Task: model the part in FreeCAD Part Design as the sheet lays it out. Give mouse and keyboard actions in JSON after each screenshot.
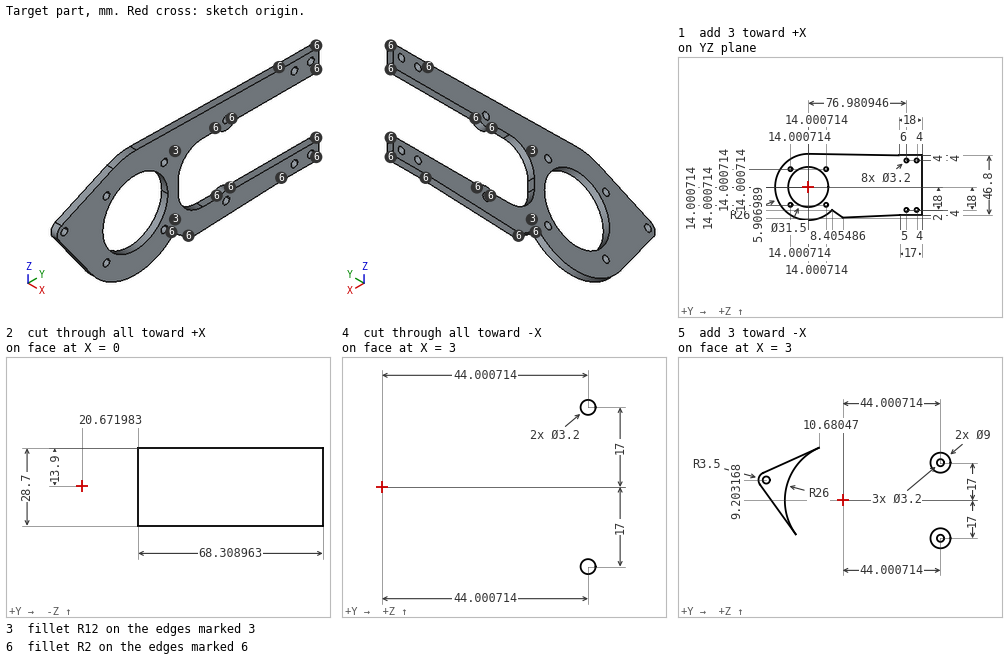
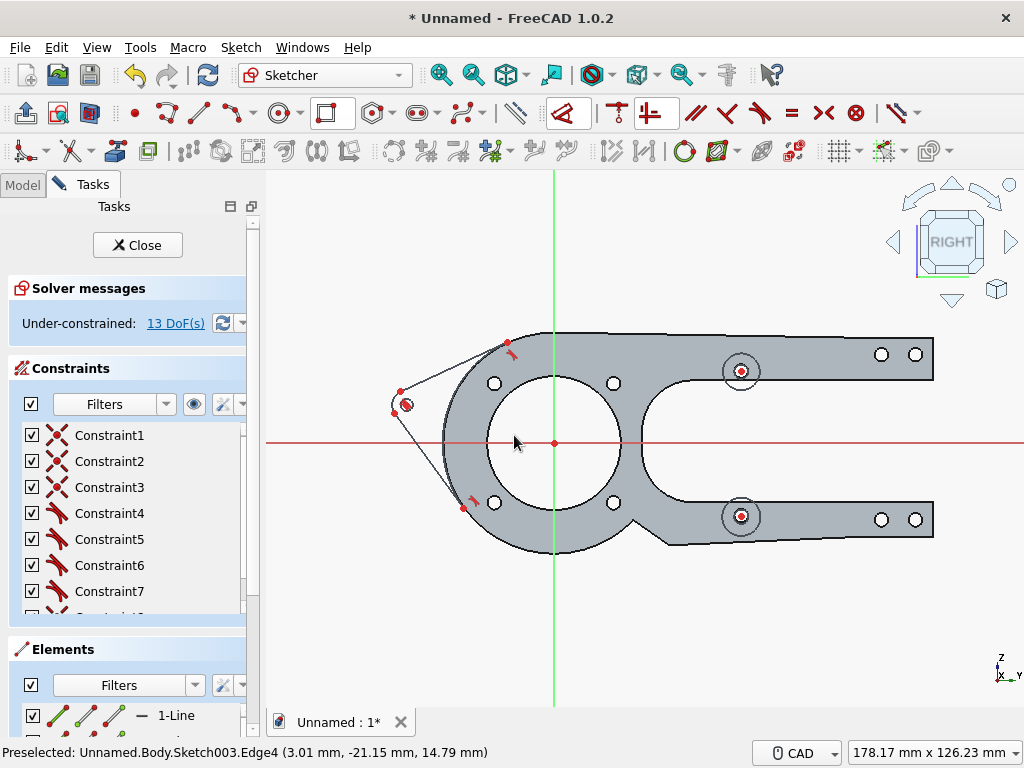
{"action": "left_click", "coordinate": [754, 359]}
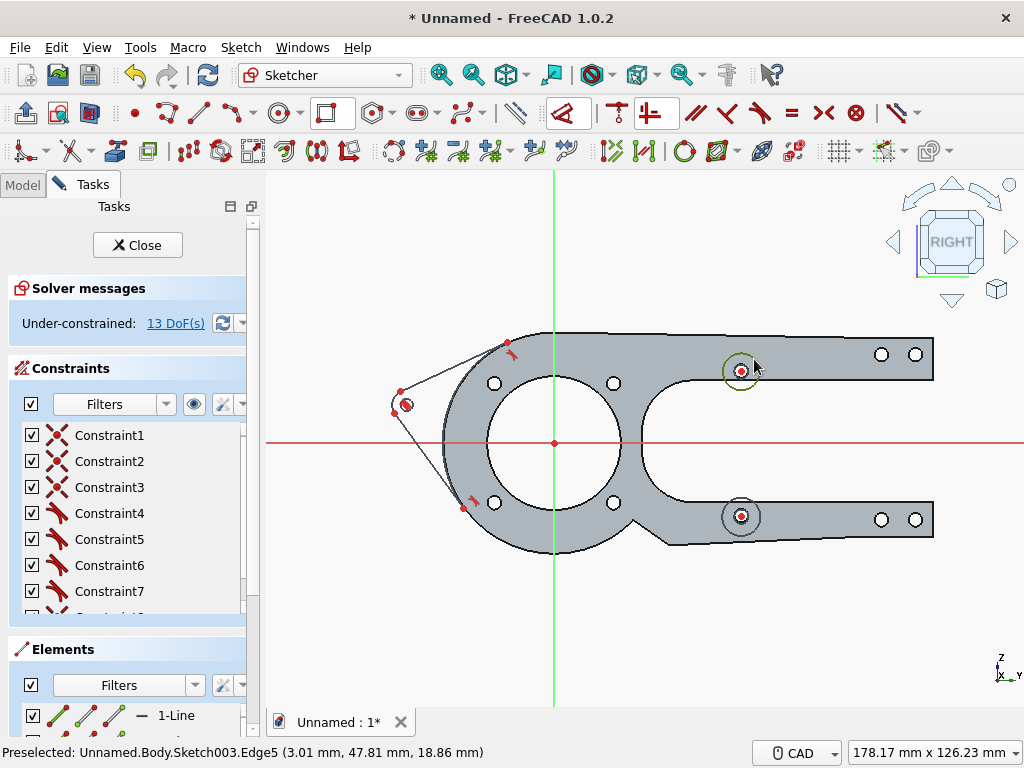
{"action": "left_click", "coordinate": [755, 503]}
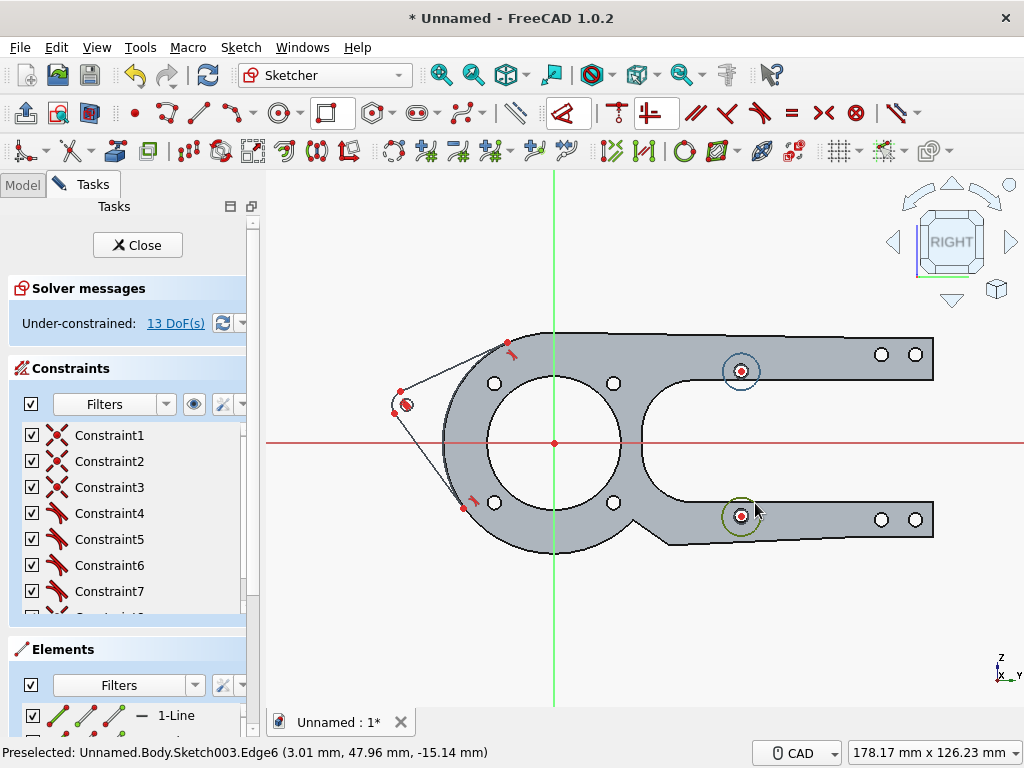
{"action": "left_click", "coordinate": [792, 114]}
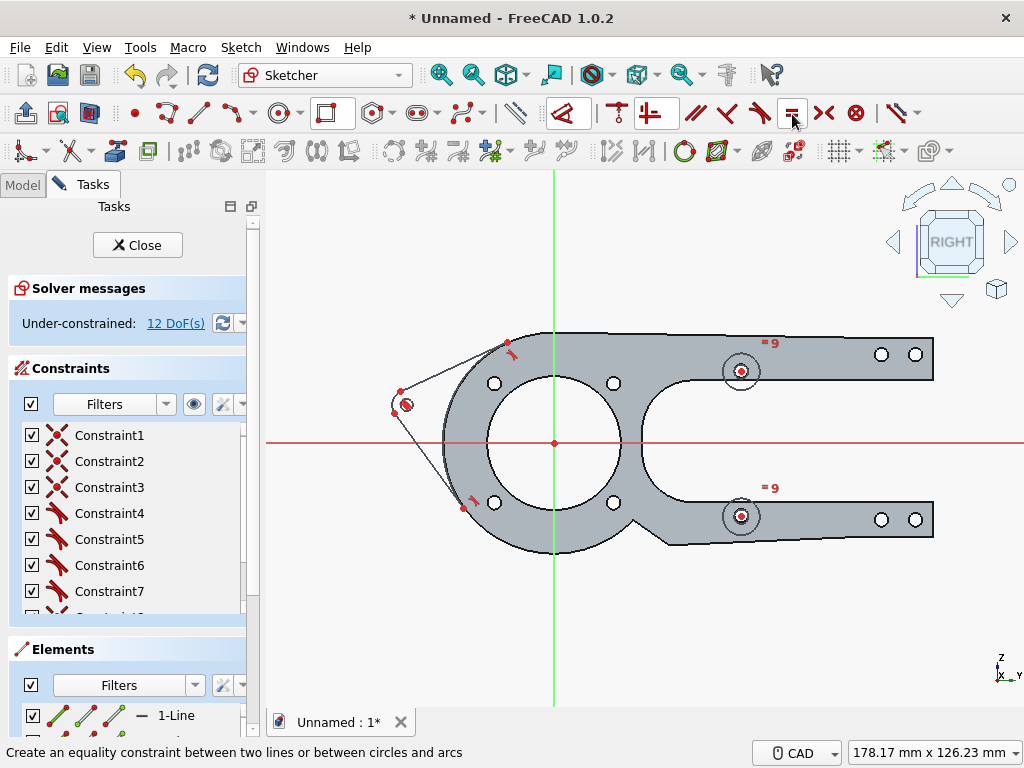
{"action": "scroll", "coordinate": [736, 367], "scroll_direction": "up", "scroll_amount": 4}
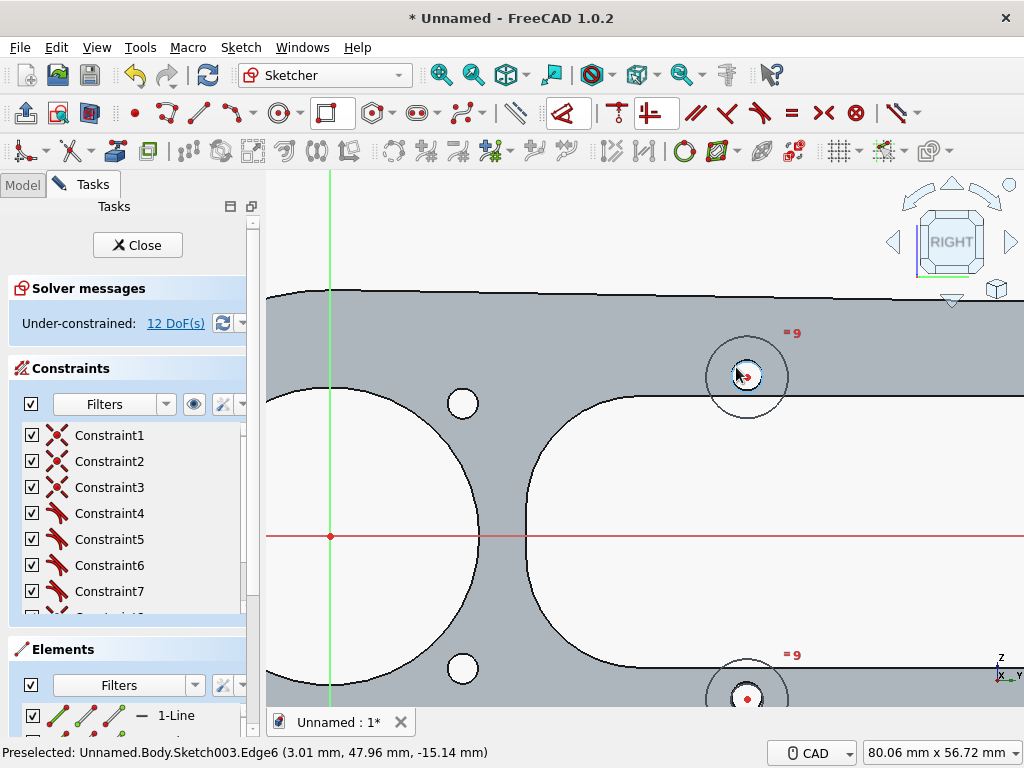
{"action": "left_click", "coordinate": [736, 366]}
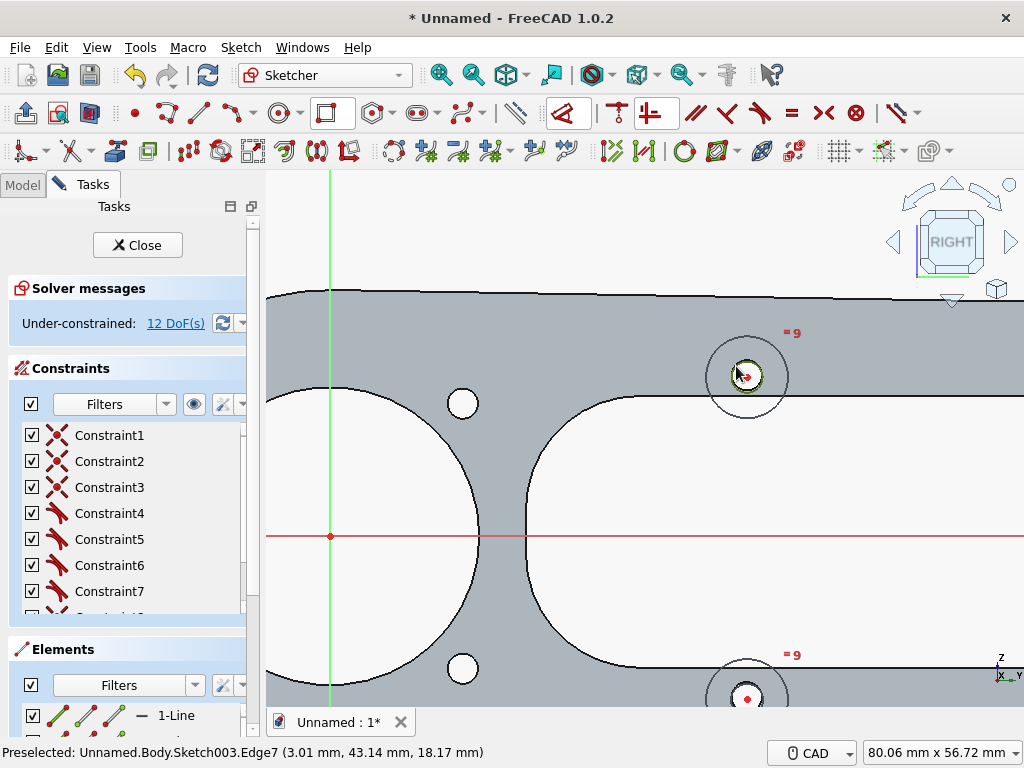
{"action": "scroll", "coordinate": [736, 367], "scroll_direction": "down", "scroll_amount": 4}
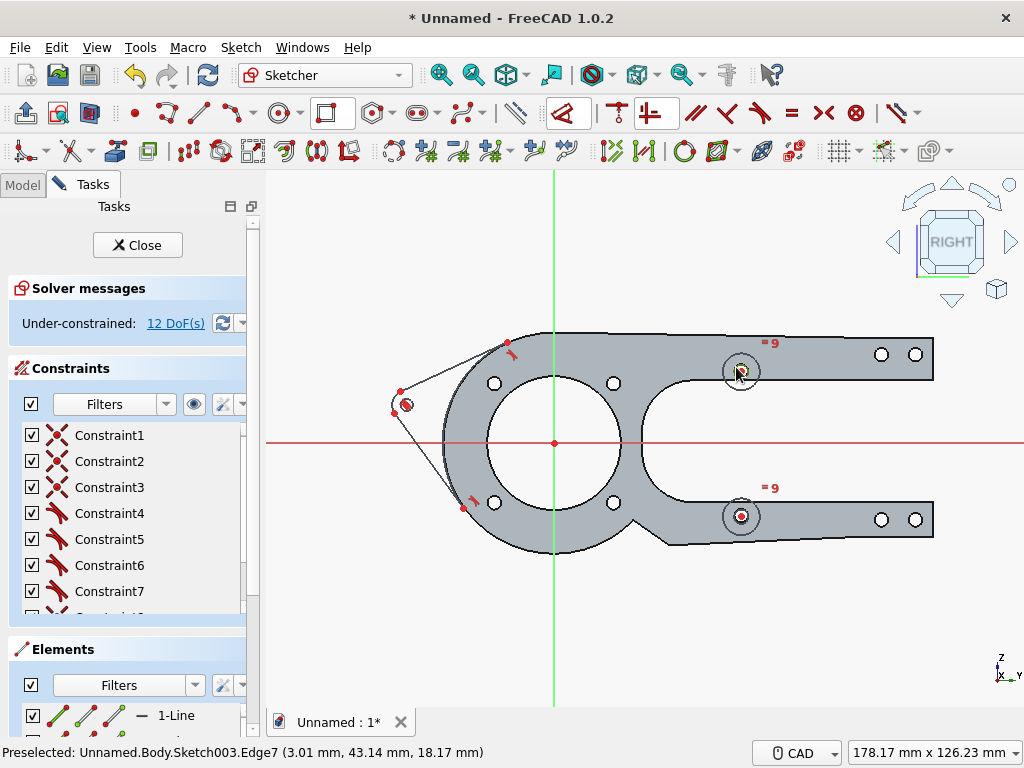
{"action": "scroll", "coordinate": [746, 512], "scroll_direction": "up", "scroll_amount": 4}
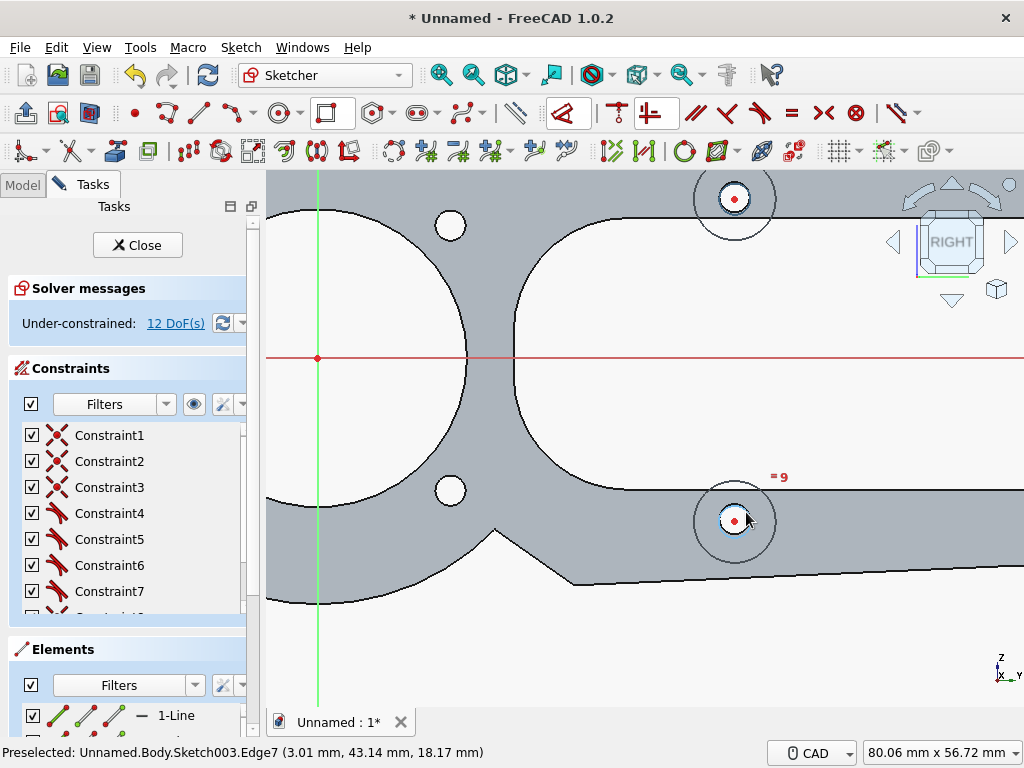
{"action": "left_click", "coordinate": [746, 511]}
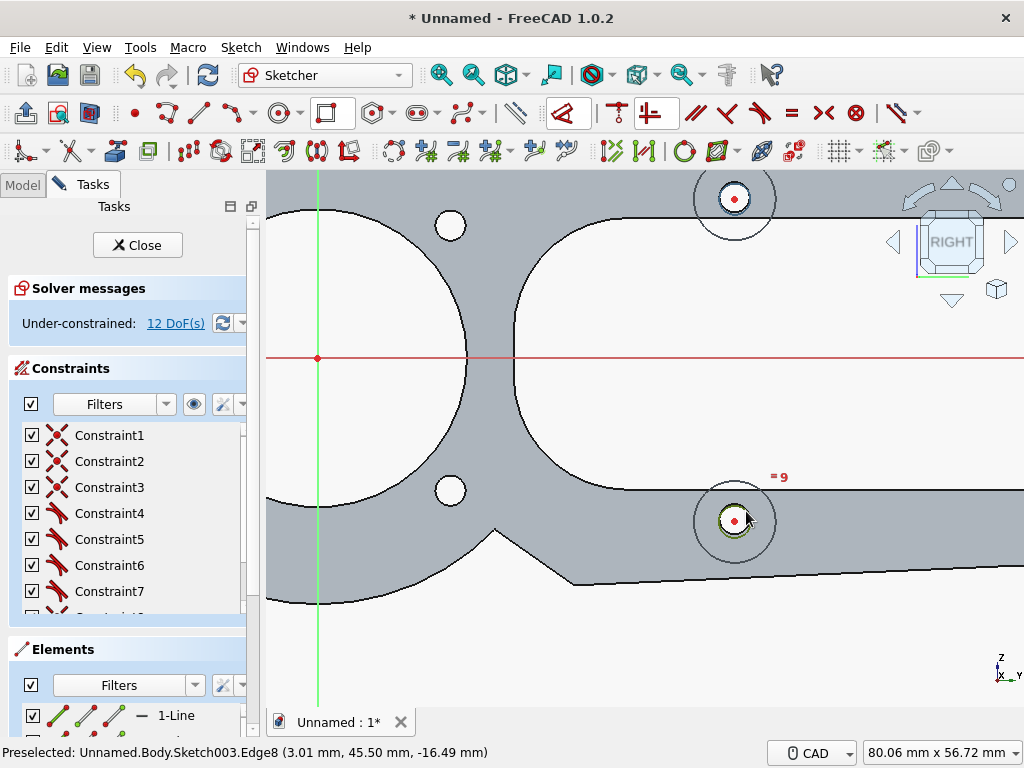
{"action": "scroll", "coordinate": [746, 513], "scroll_direction": "down", "scroll_amount": 4}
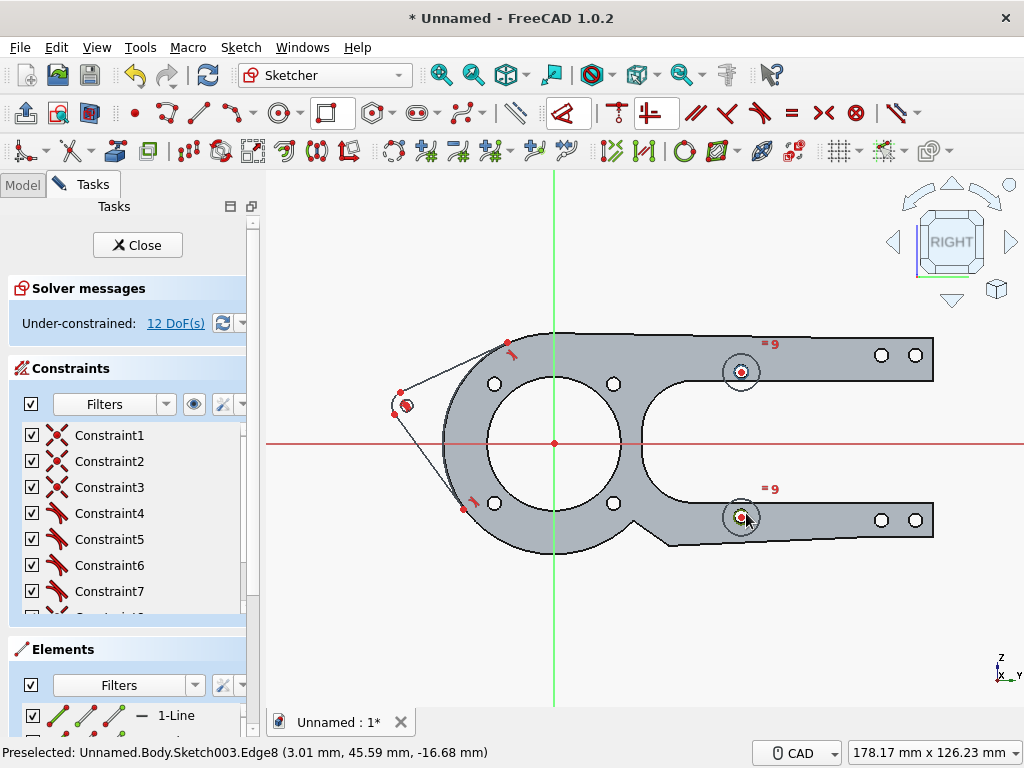
{"action": "scroll", "coordinate": [411, 401], "scroll_direction": "up", "scroll_amount": 5}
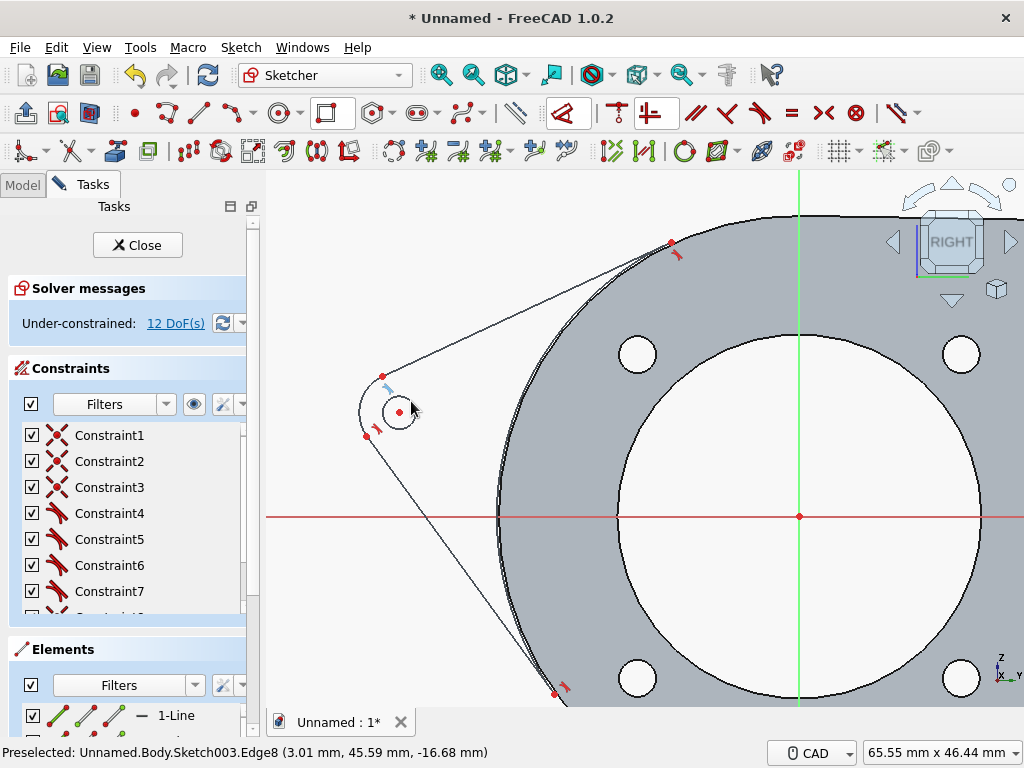
{"action": "left_click", "coordinate": [411, 401]}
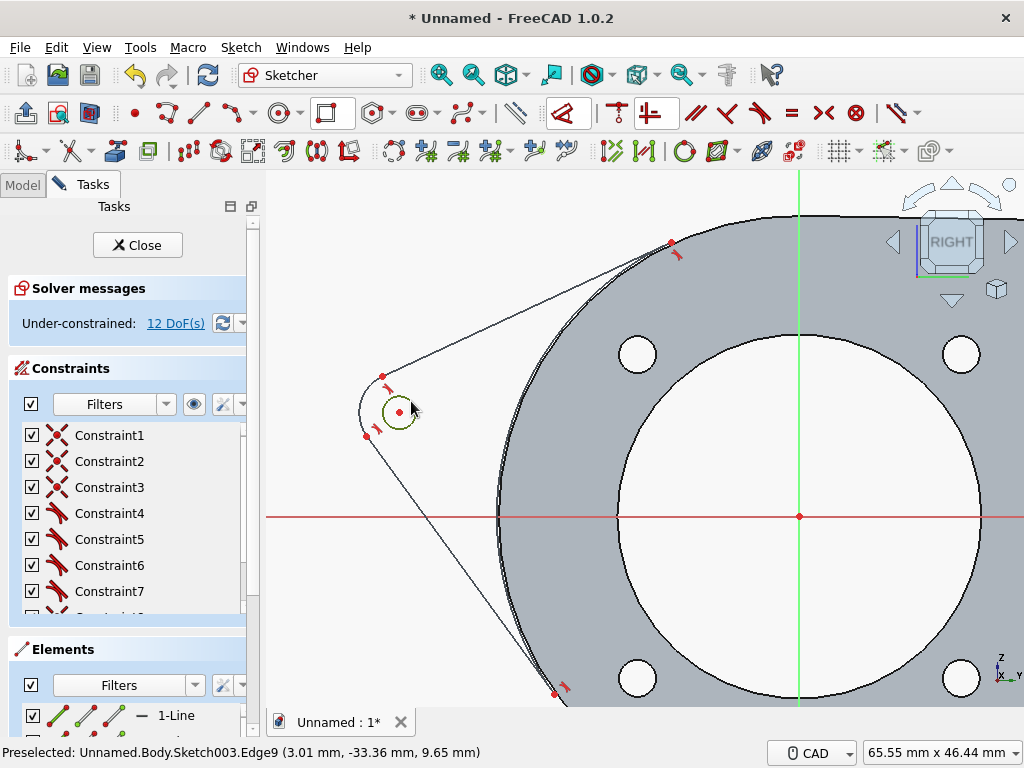
{"action": "left_click", "coordinate": [792, 114]}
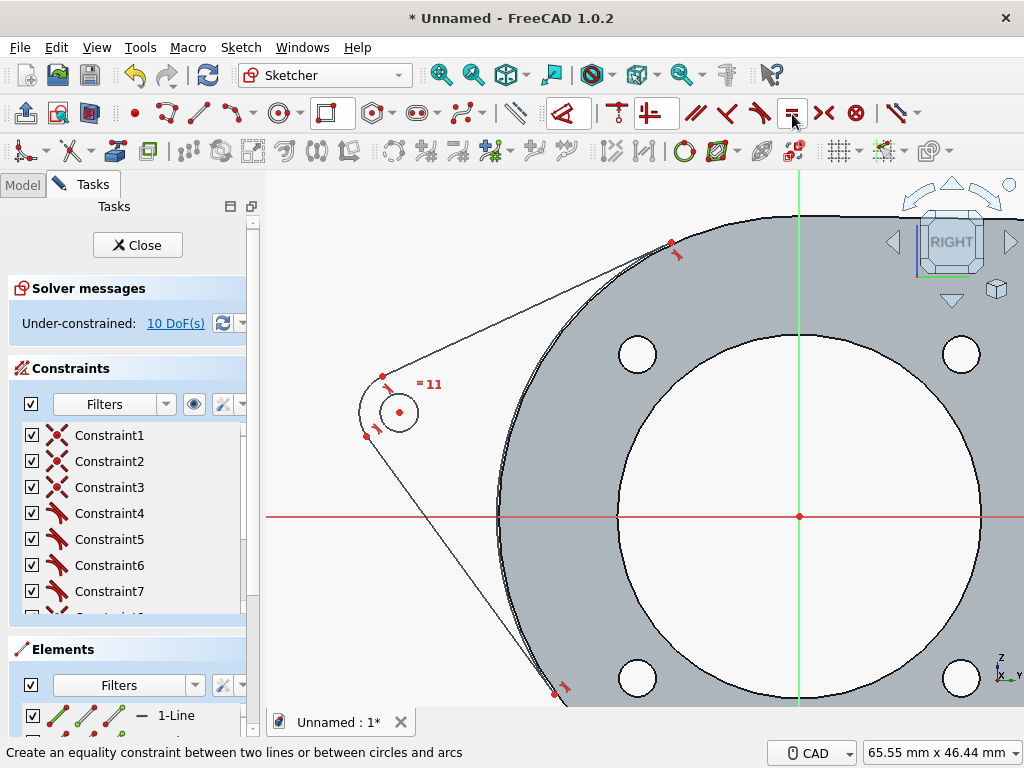
{"action": "left_click", "coordinate": [366, 390]}